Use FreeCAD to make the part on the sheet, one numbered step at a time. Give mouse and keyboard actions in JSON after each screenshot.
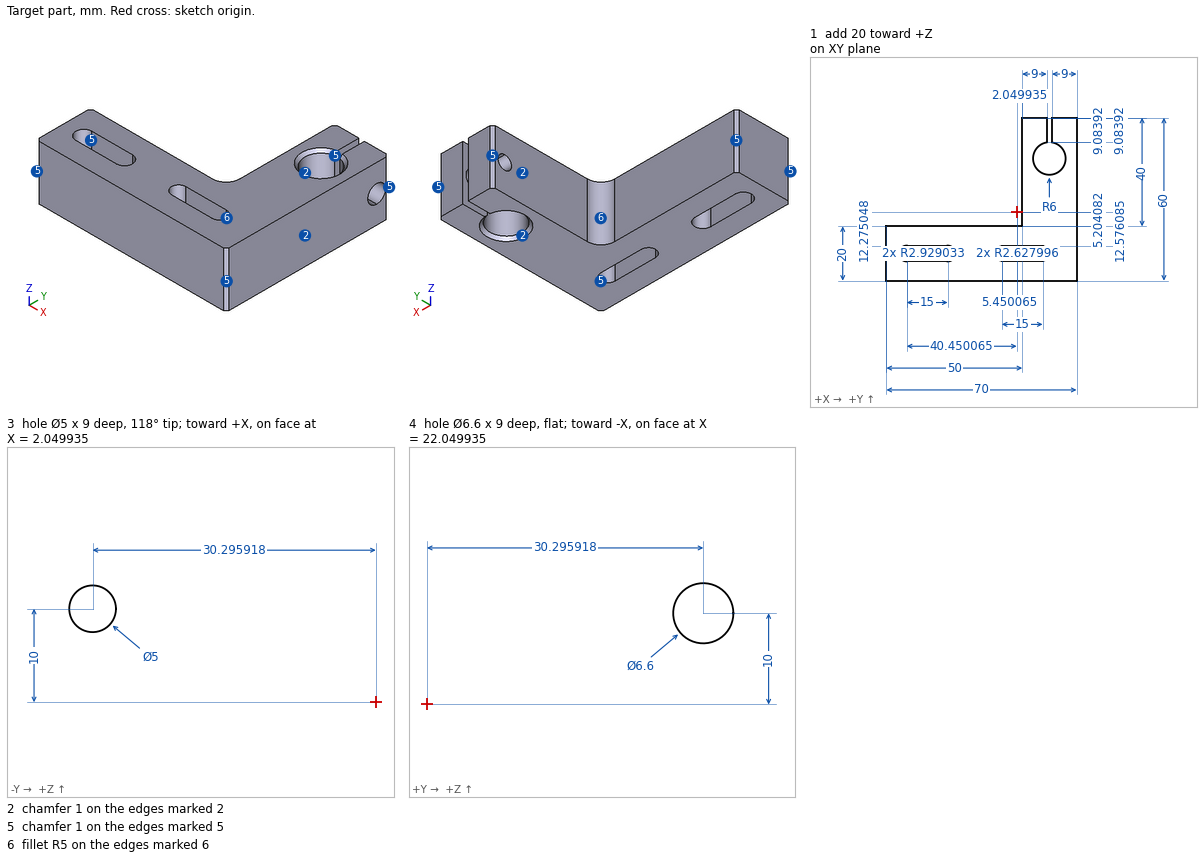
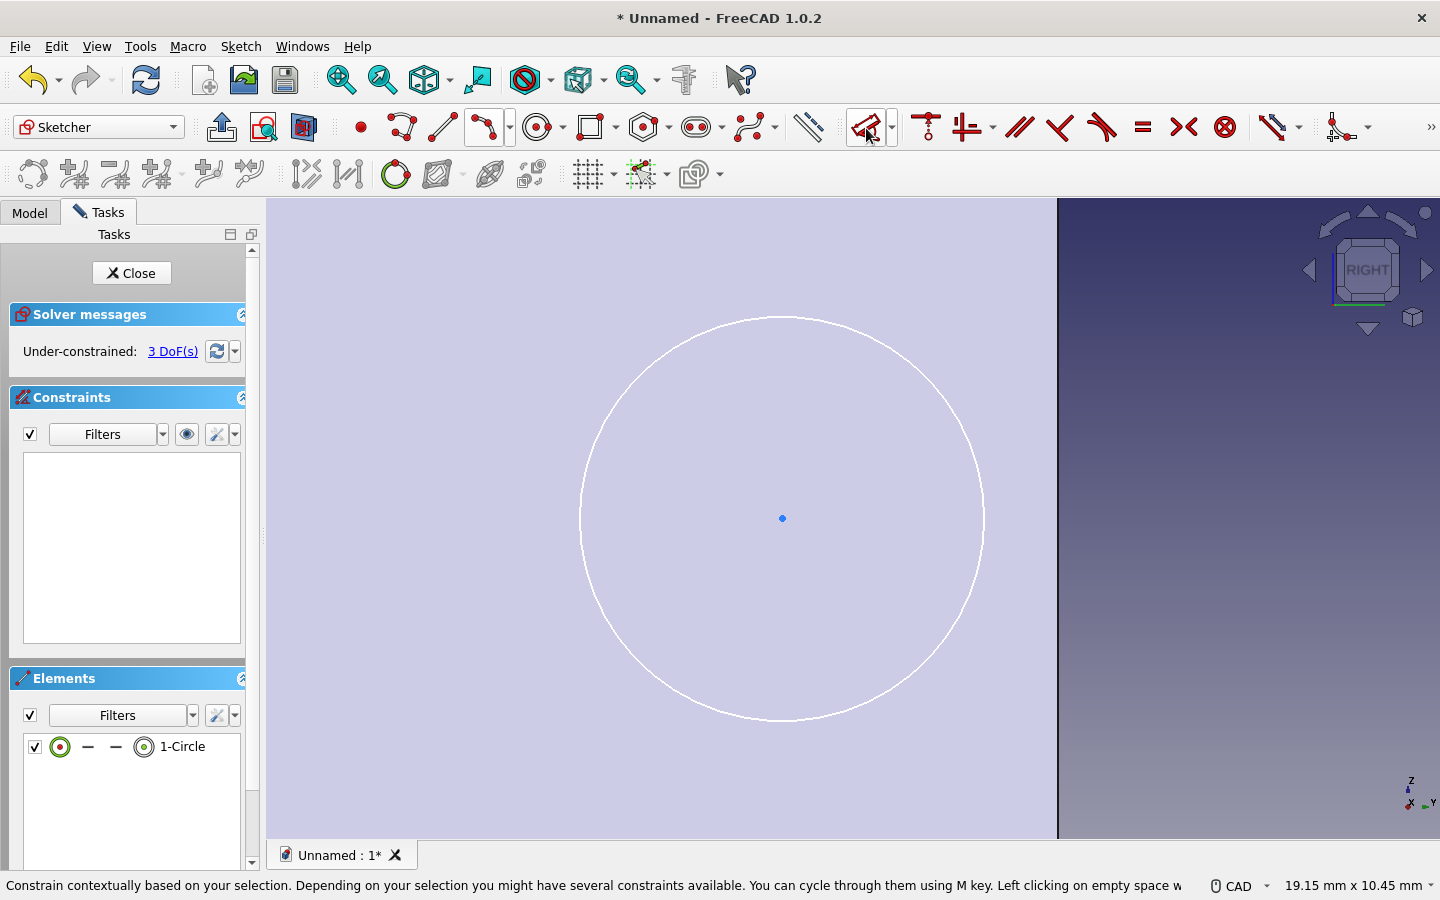
{"action": "left_click", "coordinate": [925, 376]}
{"action": "left_click", "coordinate": [948, 353]}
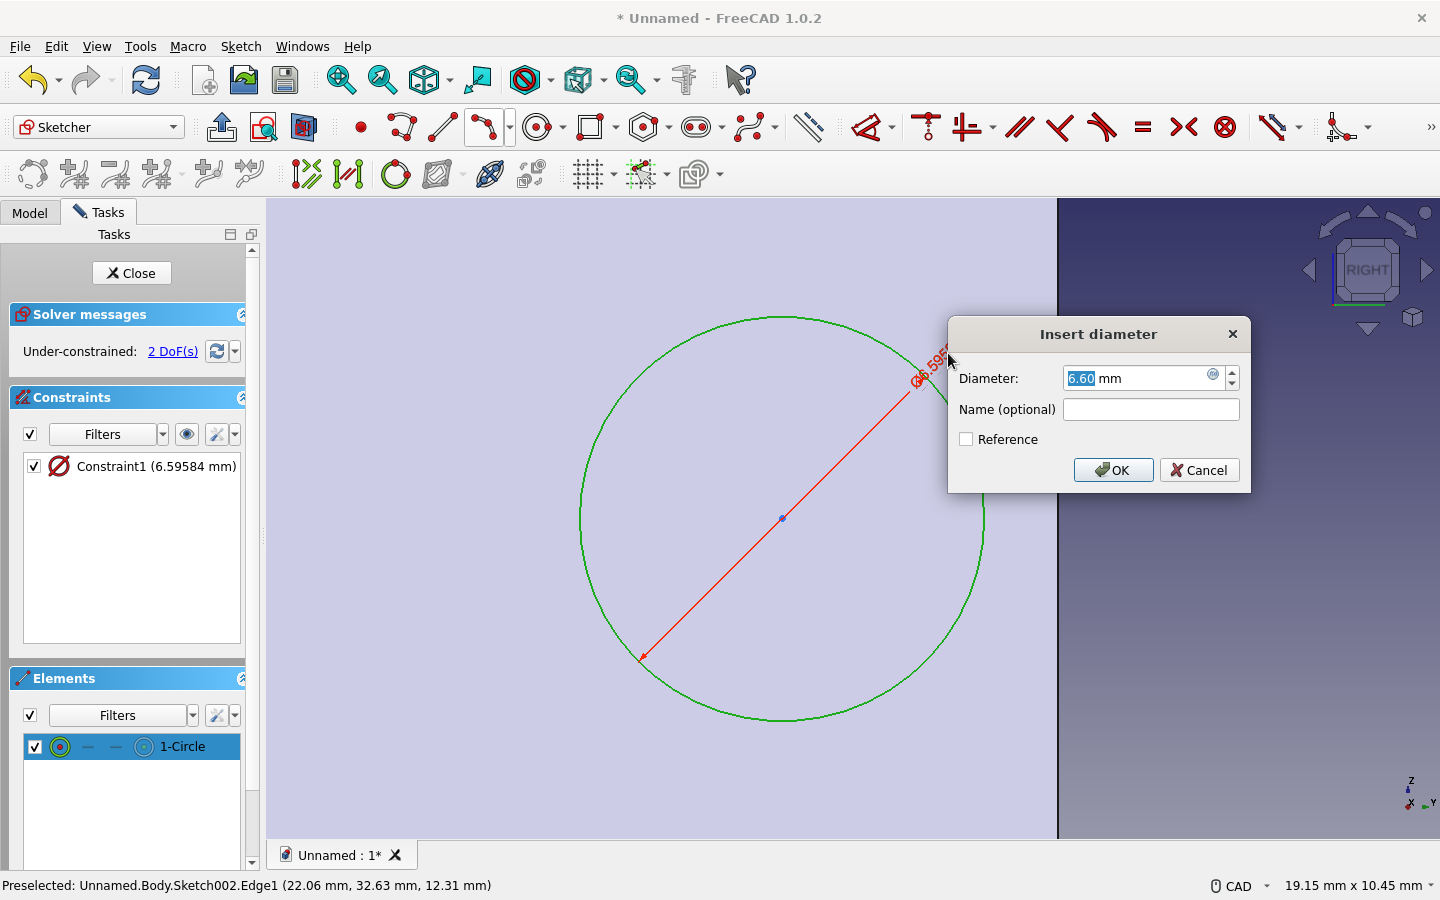
{"action": "type", "text": "6.6"}
{"action": "key", "text": "Return"}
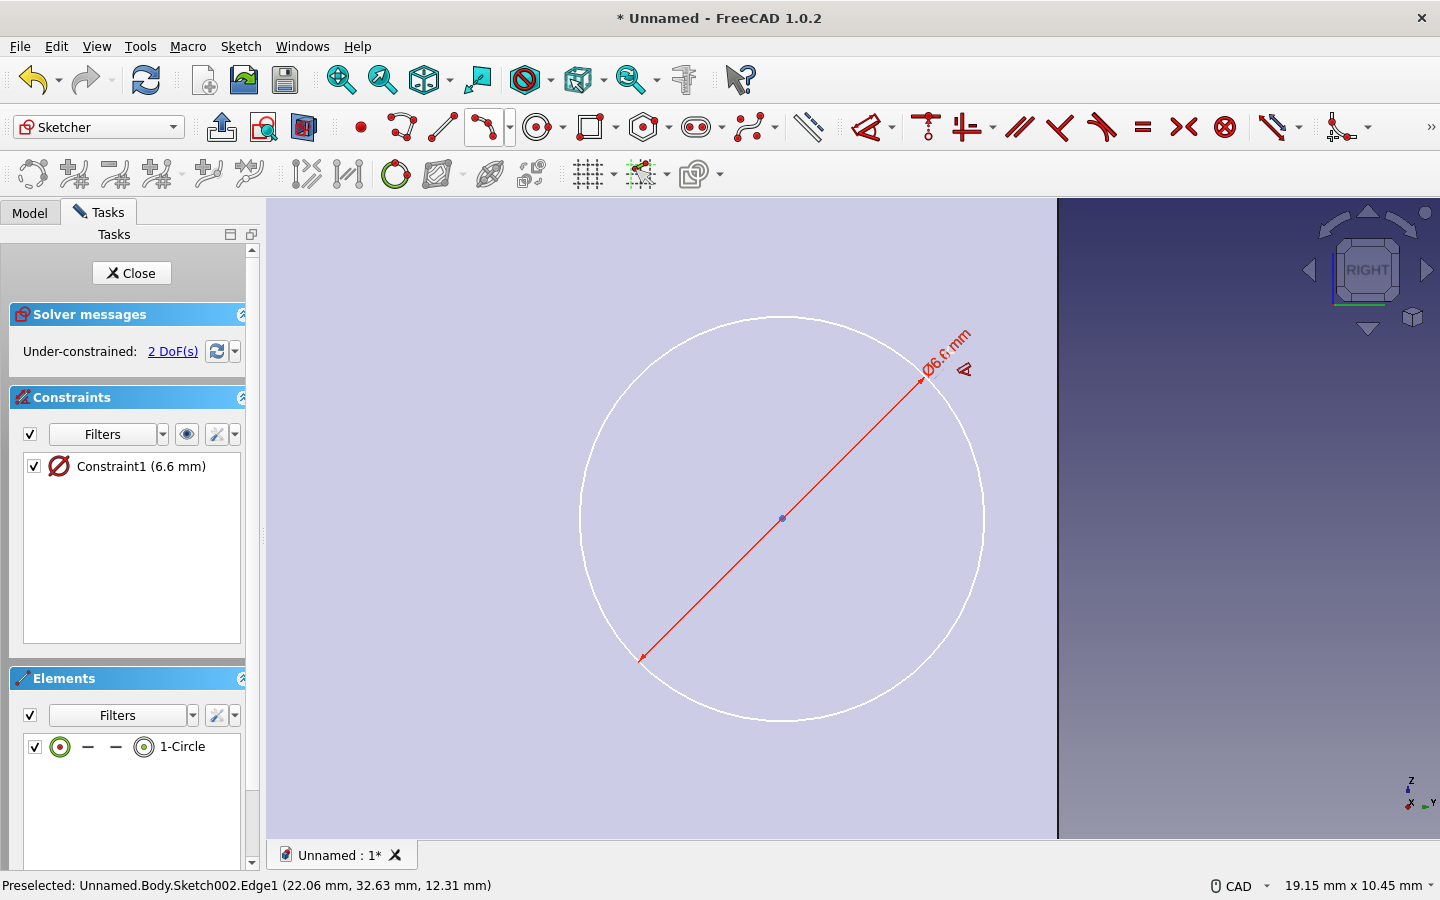
{"action": "left_click", "coordinate": [782, 519]}
{"action": "left_click", "coordinate": [816, 665]}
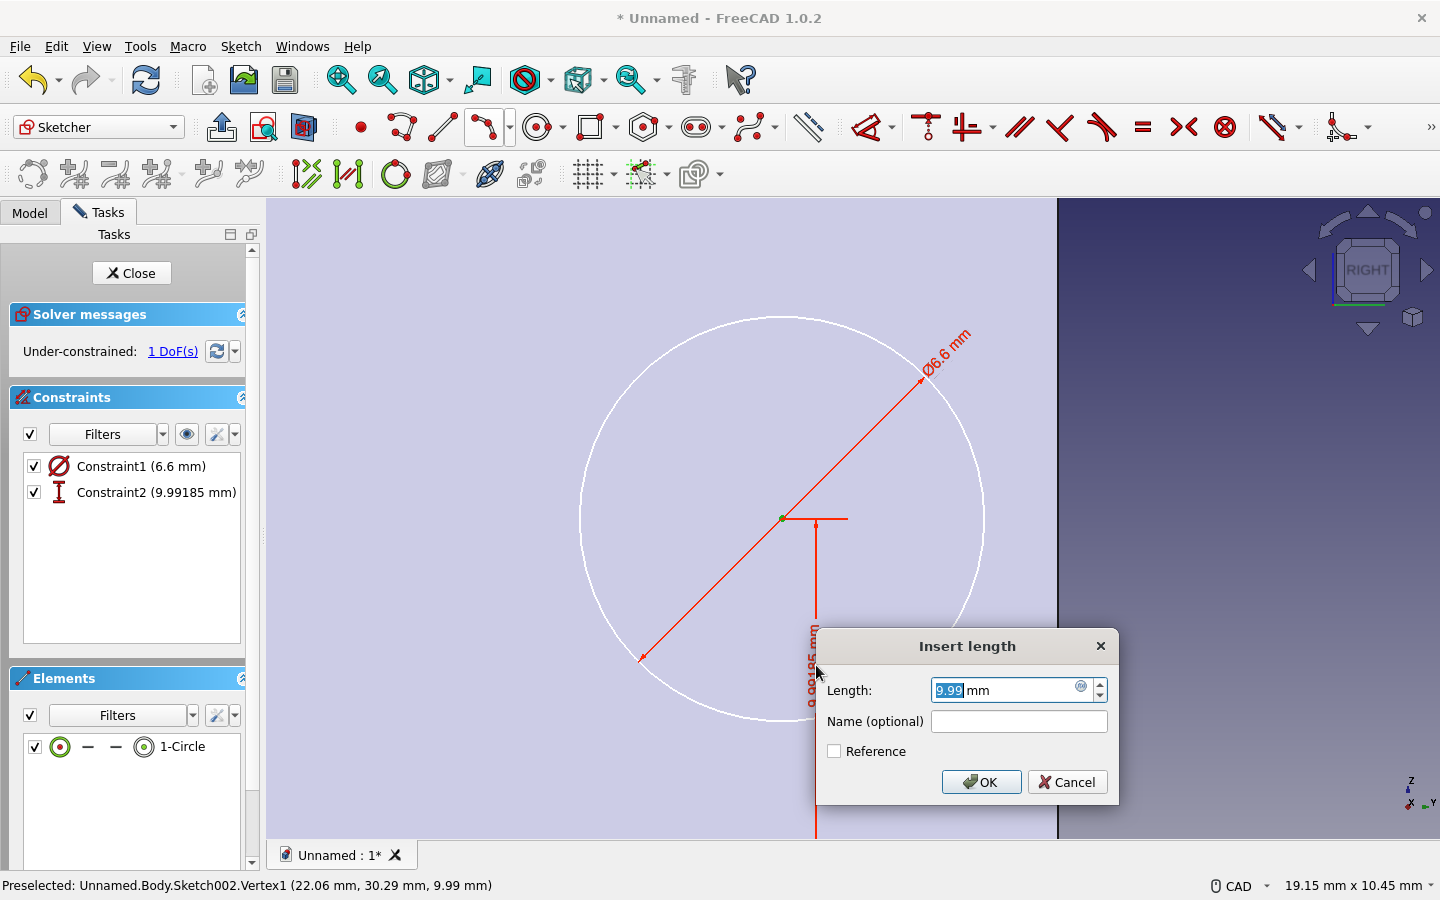
{"action": "type", "text": "10"}
{"action": "key", "text": "Return"}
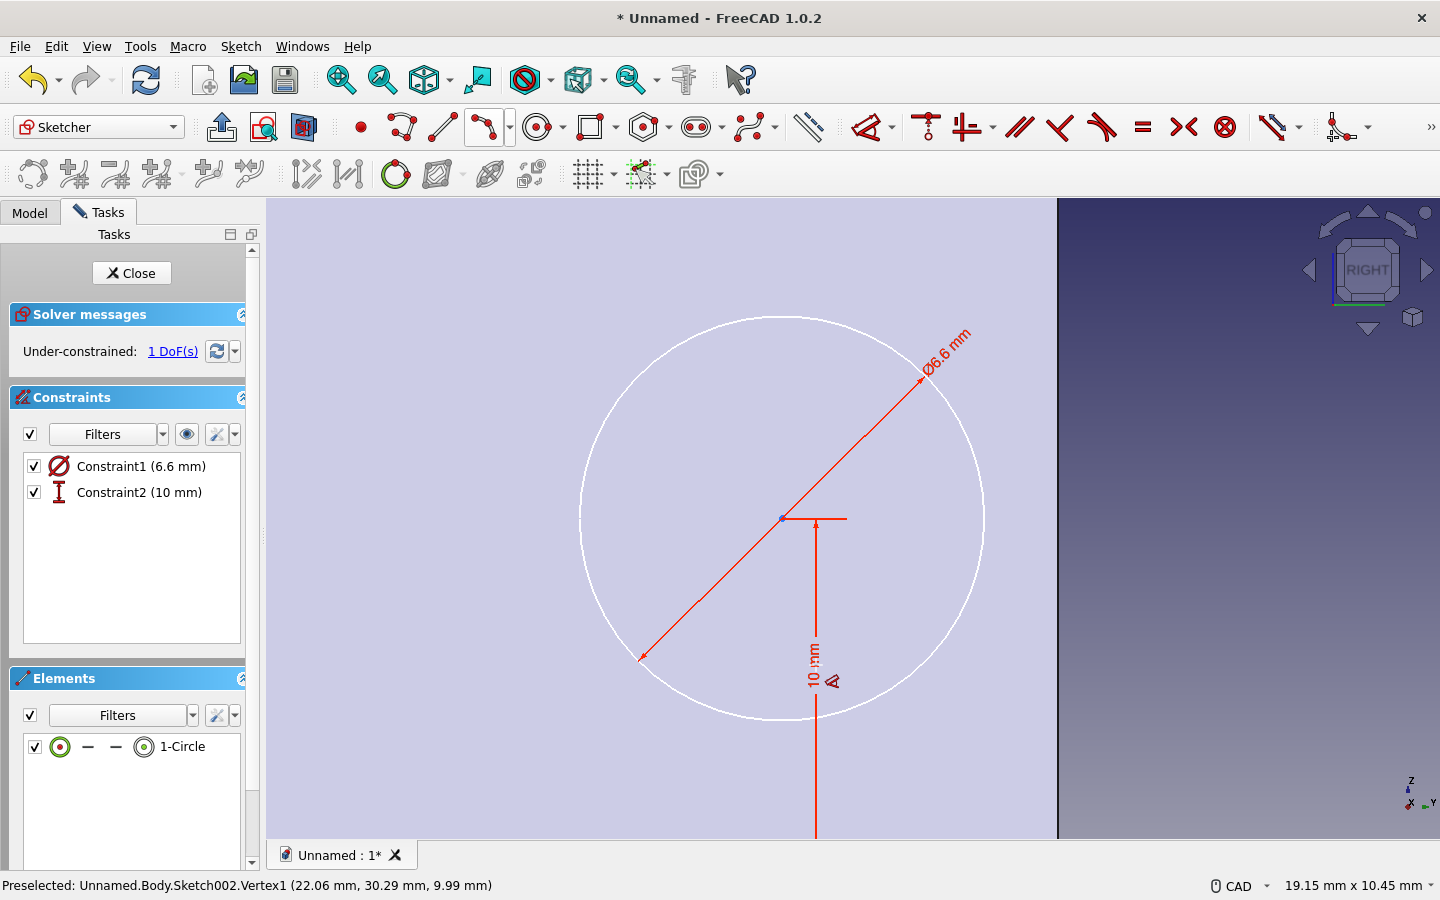
{"action": "left_click", "coordinate": [782, 518]}
{"action": "left_click", "coordinate": [538, 484]}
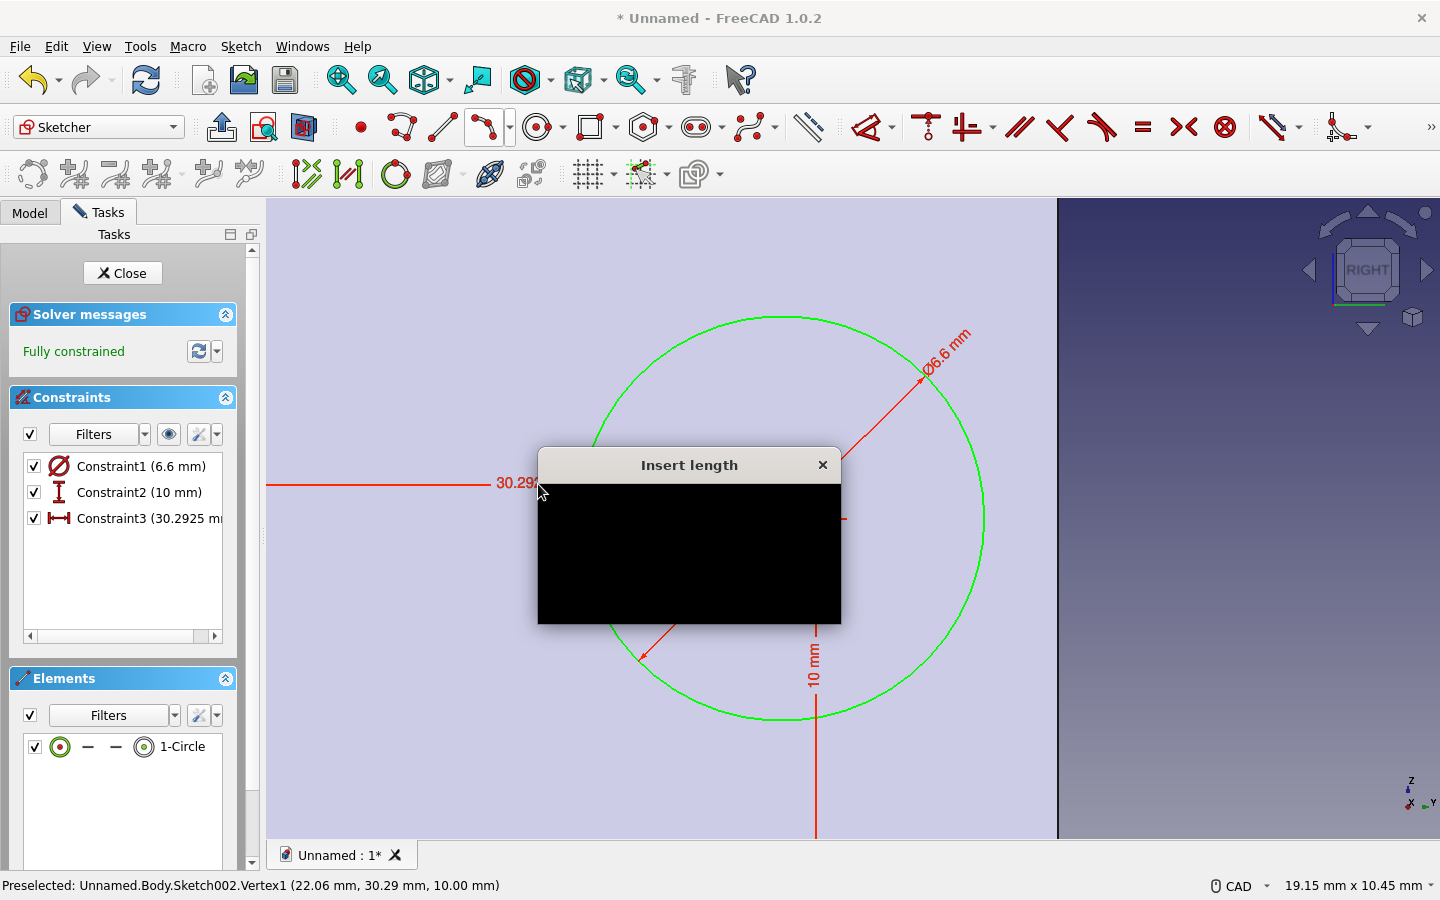
{"action": "type", "text": "30.295918"}
{"action": "key", "text": "Return"}
{"action": "key", "text": "Escape"}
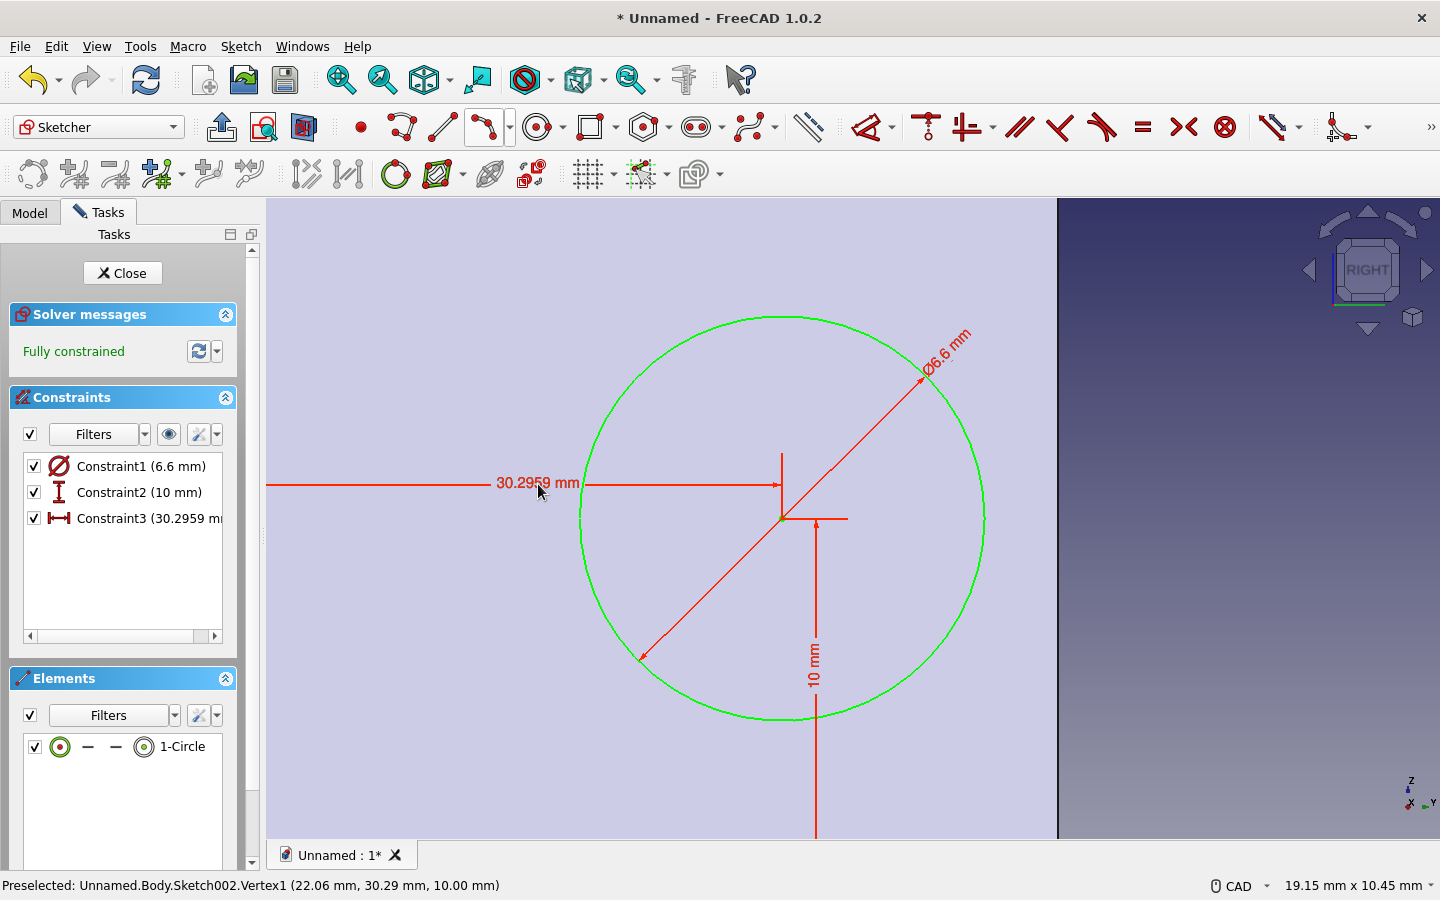
{"action": "left_click", "coordinate": [123, 273]}